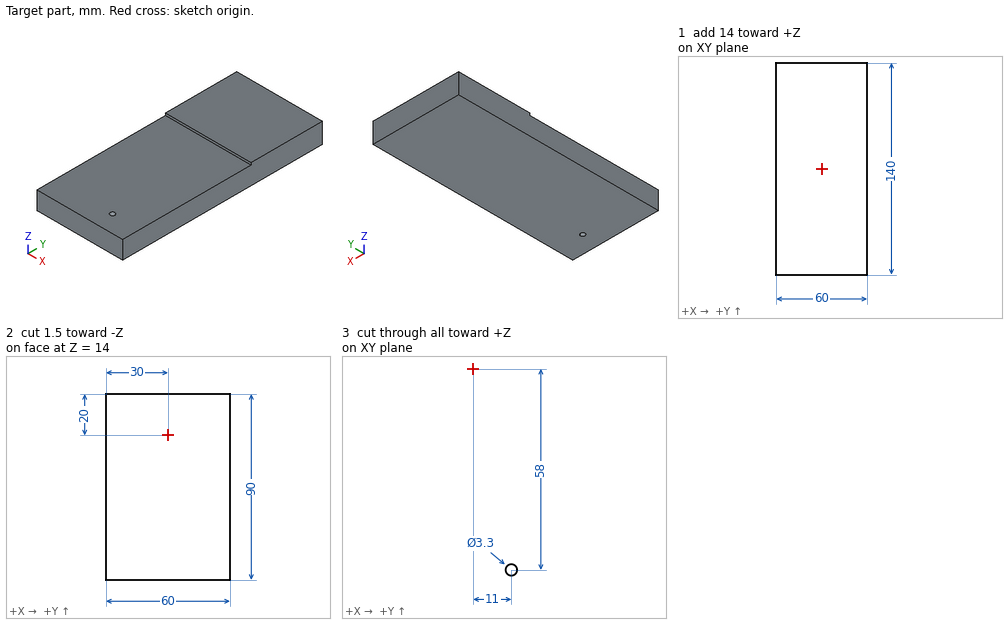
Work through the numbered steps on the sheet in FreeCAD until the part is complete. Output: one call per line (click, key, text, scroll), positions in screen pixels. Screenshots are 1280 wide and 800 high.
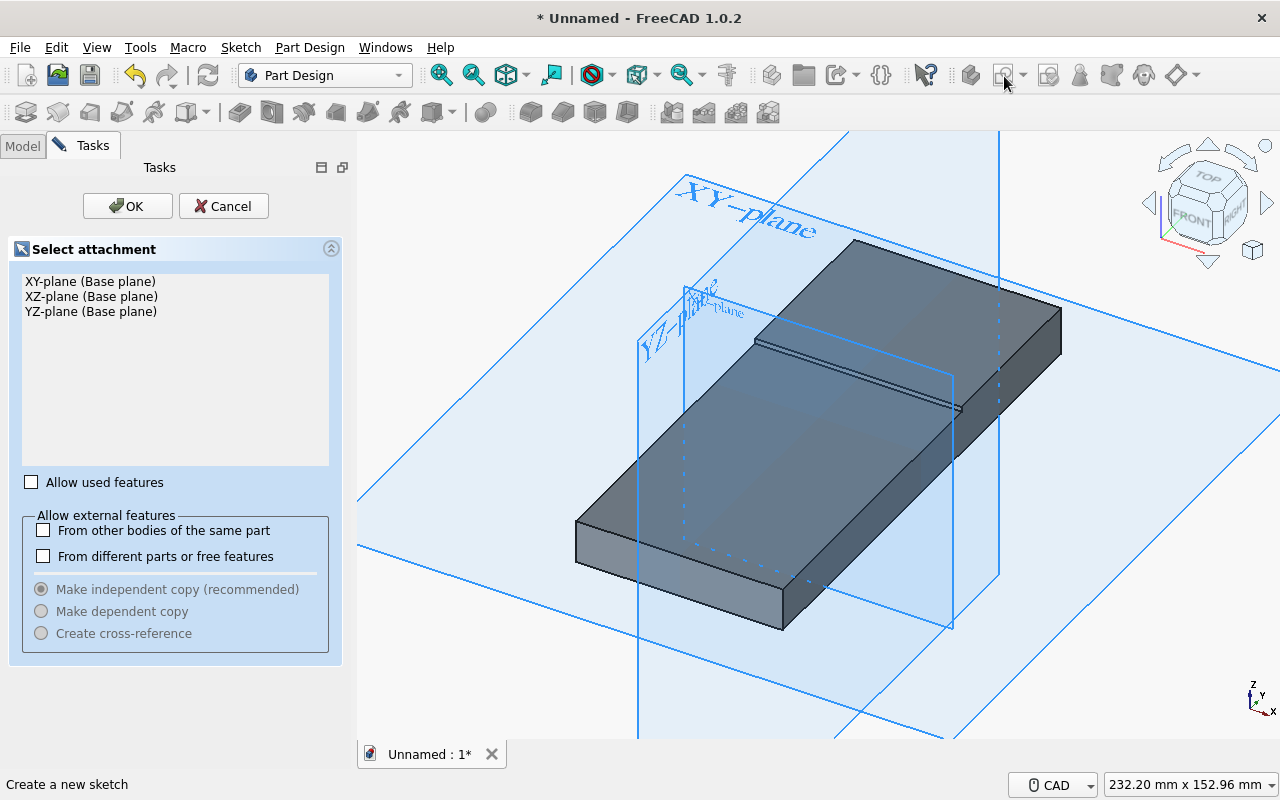
click(82, 282)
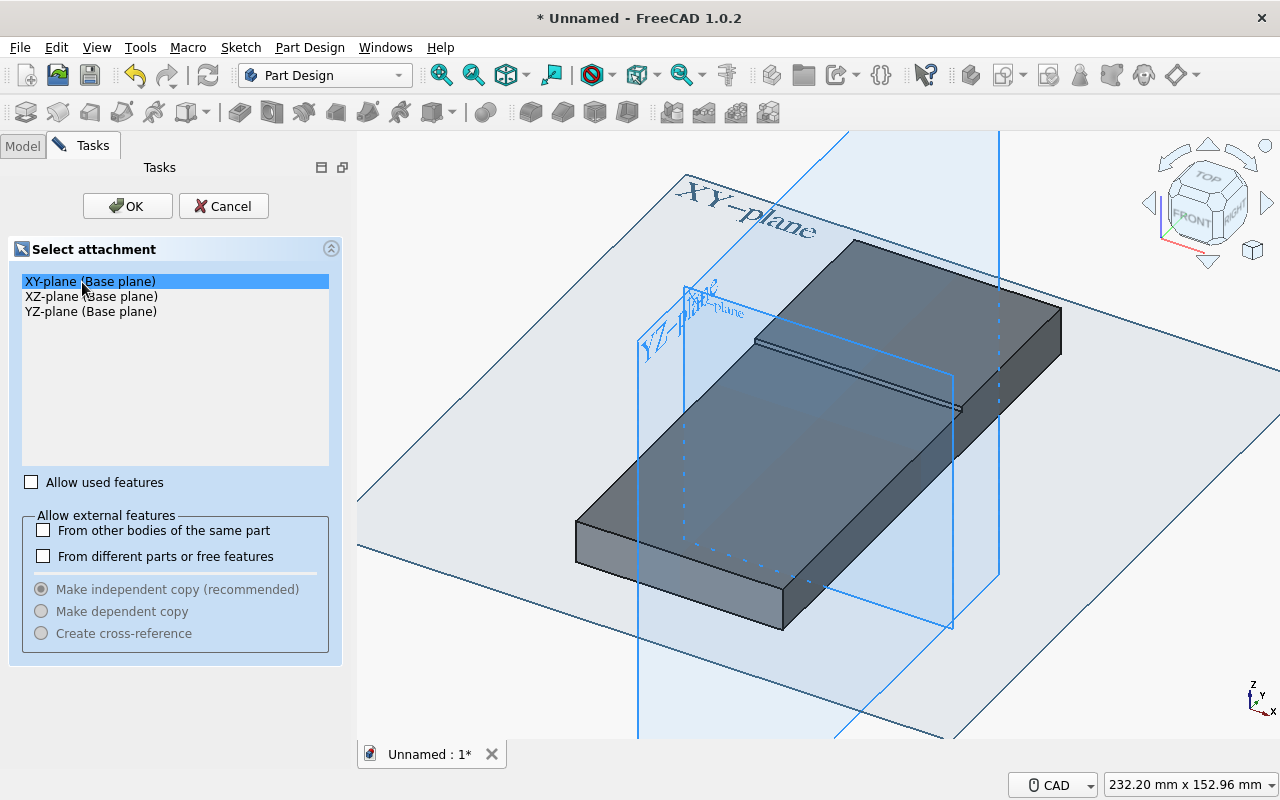
click(128, 206)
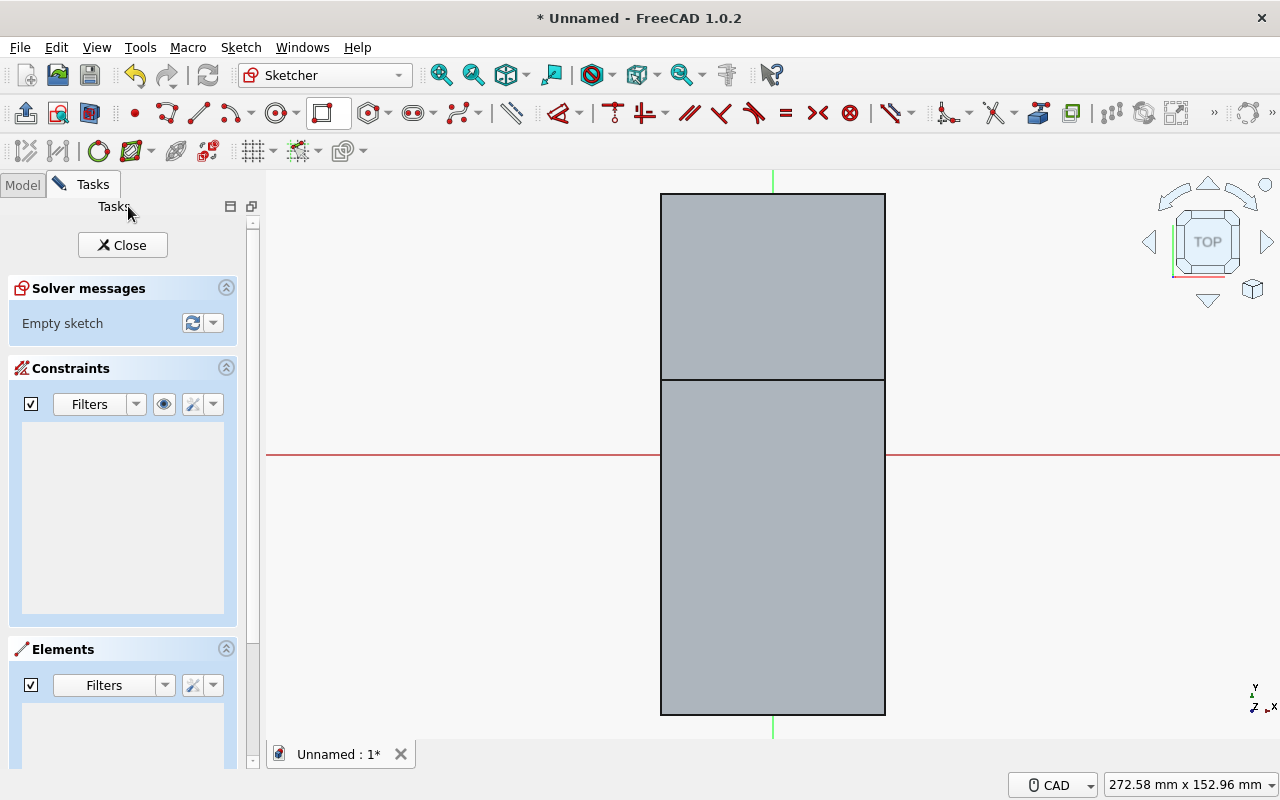
click(90, 114)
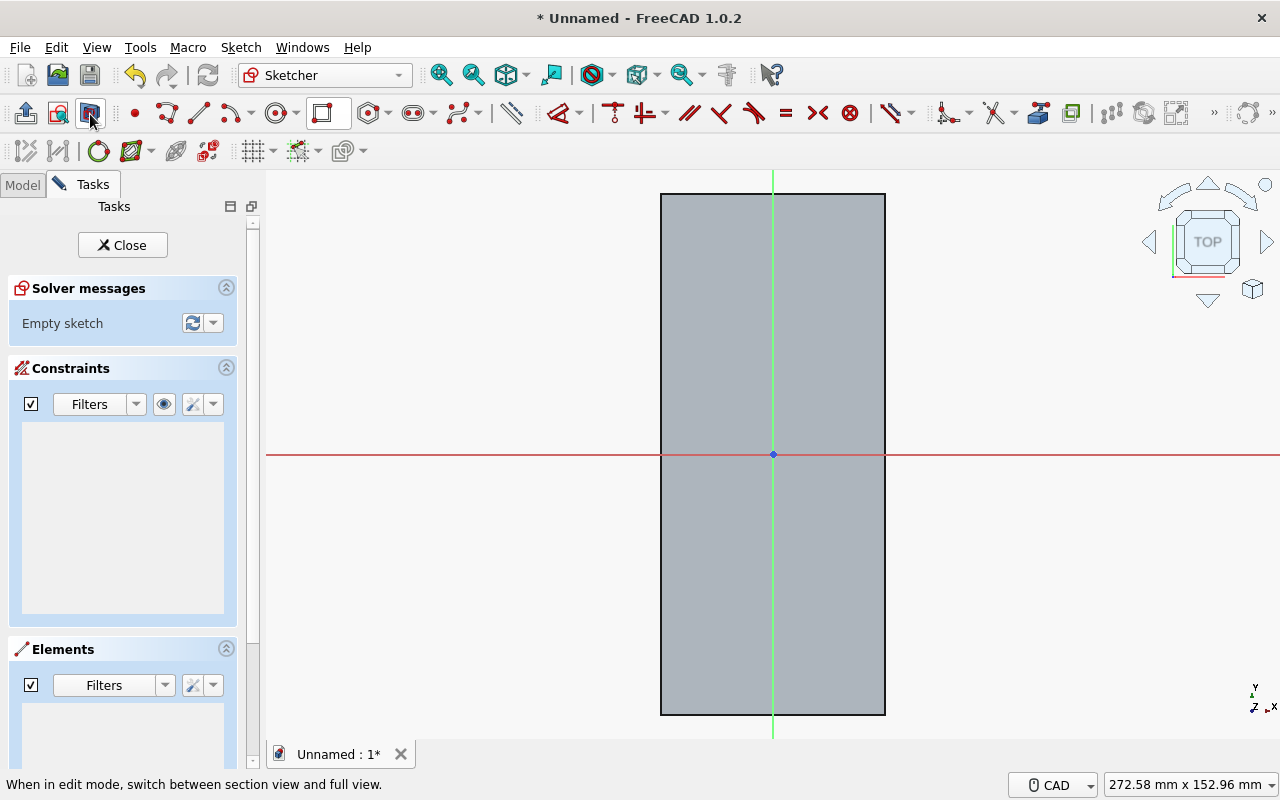
scroll(820, 682, up, 15)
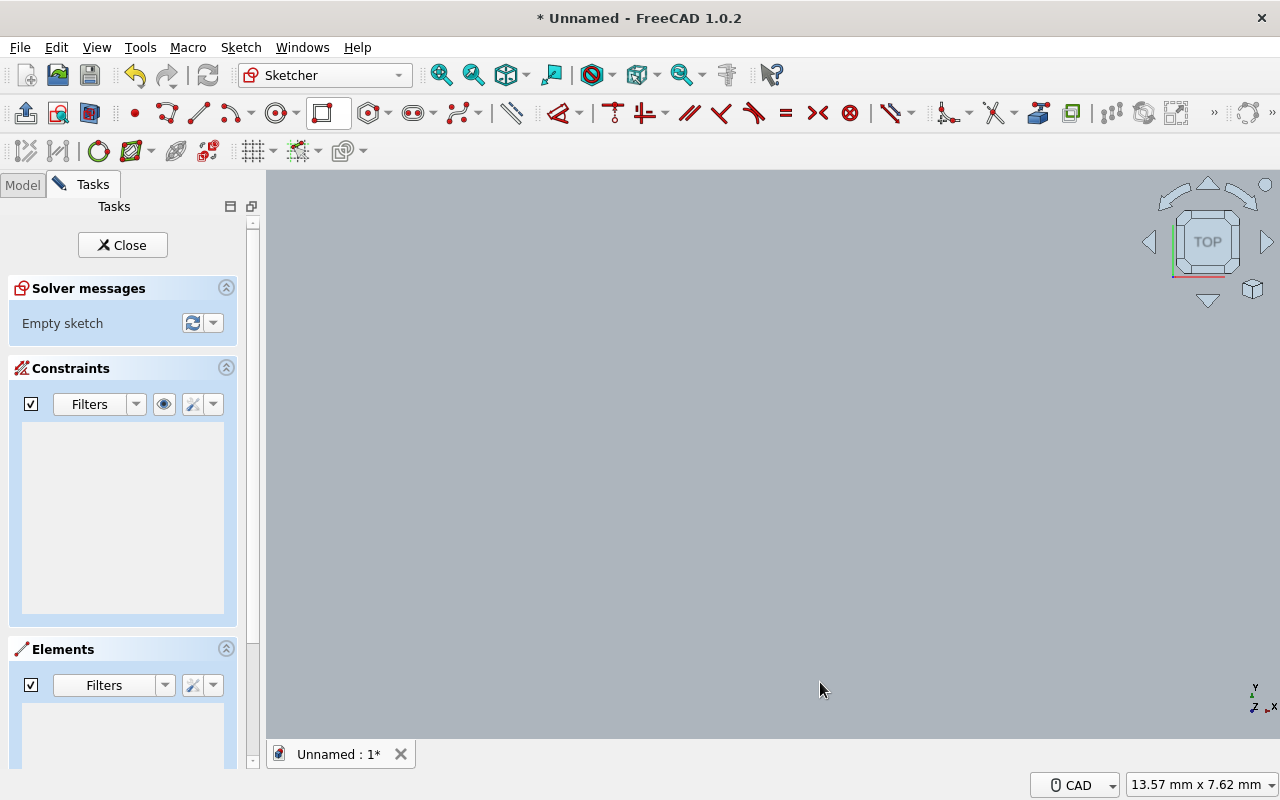
scroll(653, 377, up, 2)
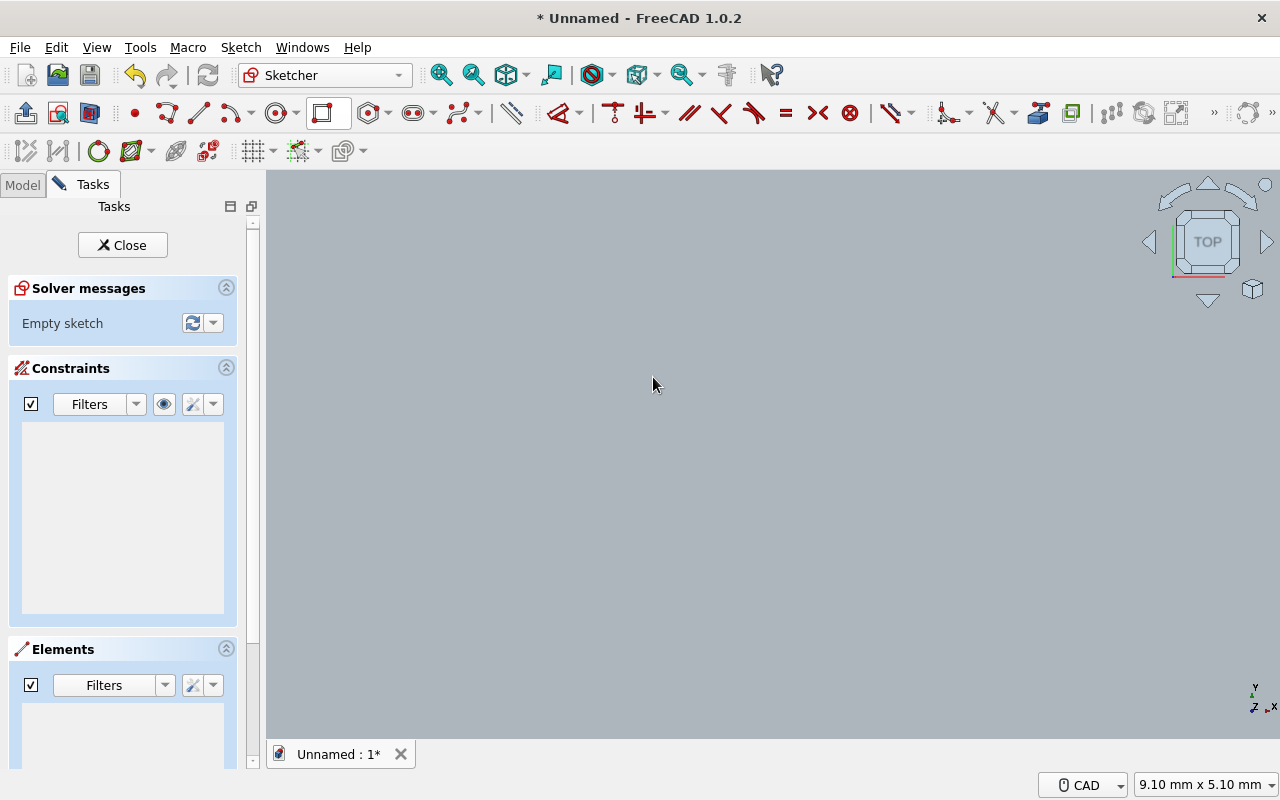
click(276, 114)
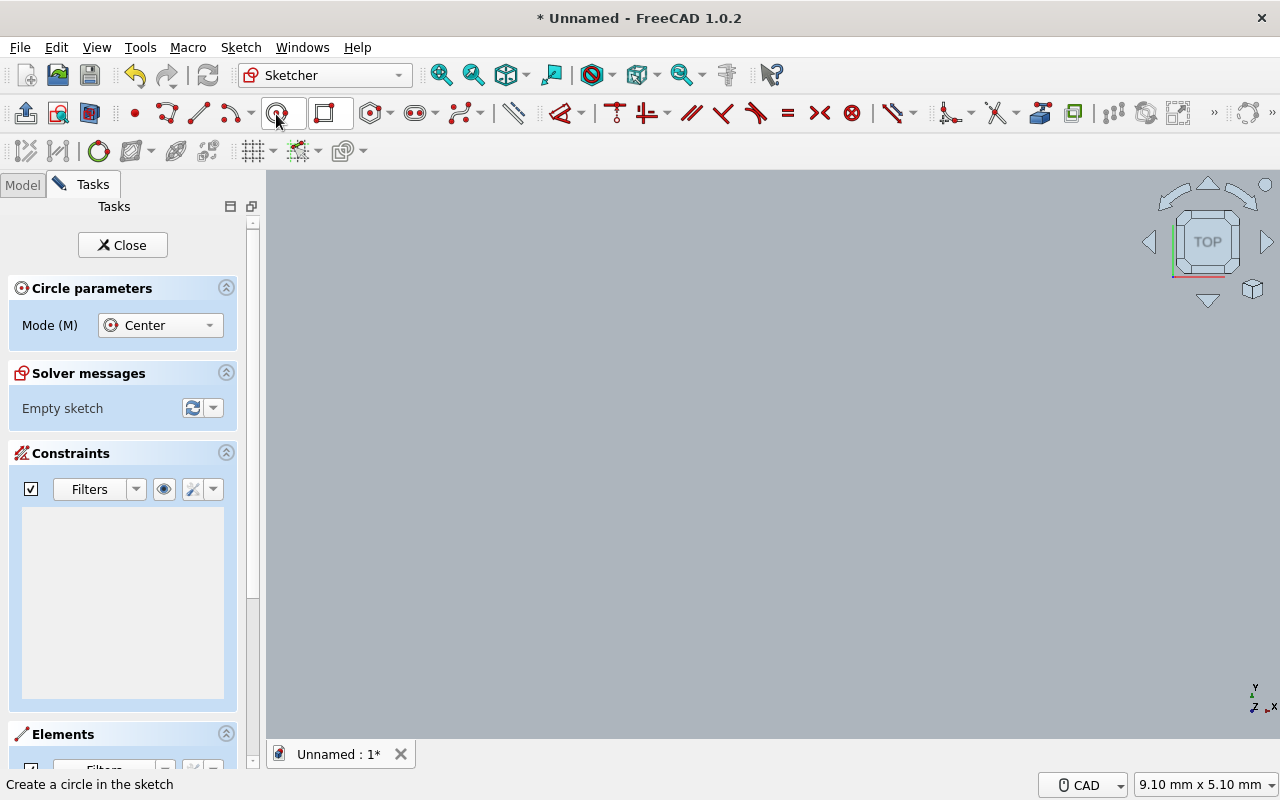
click(704, 454)
move(834, 324)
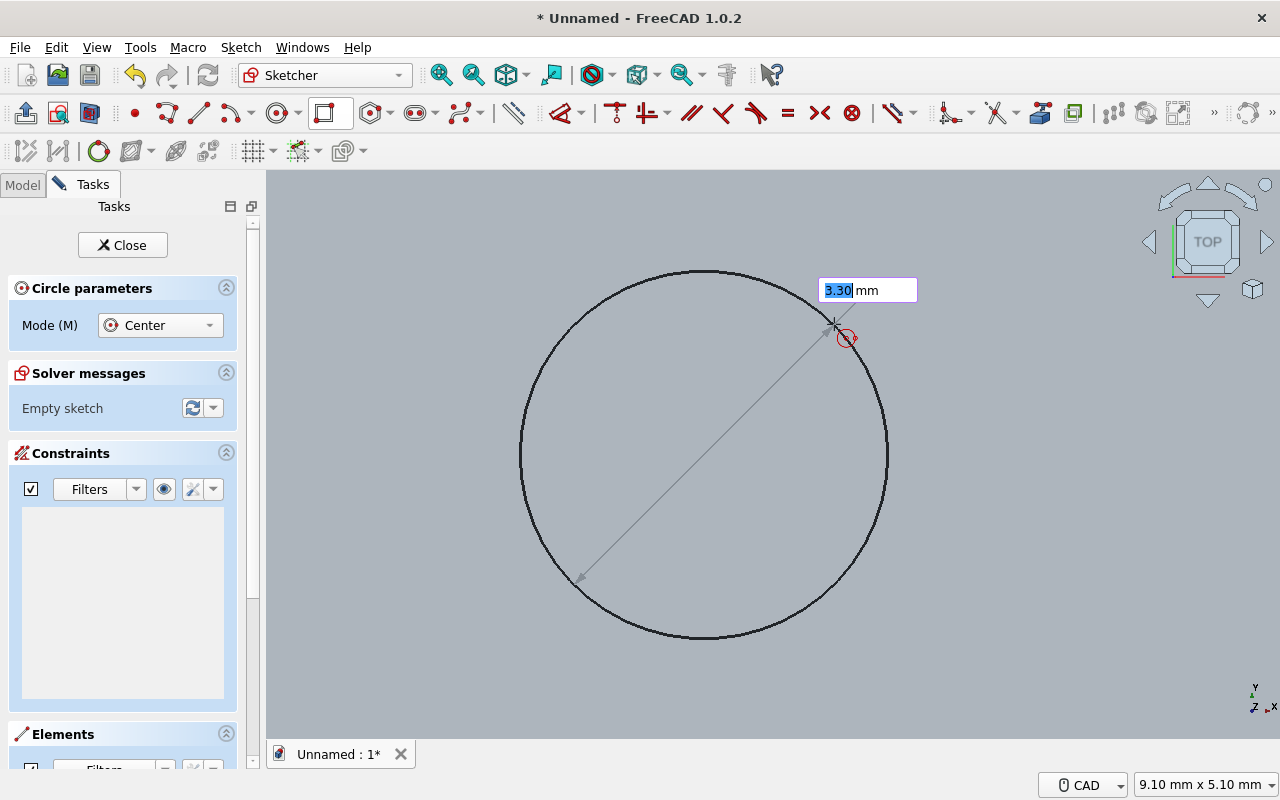
text(3.3)
key(Return)
key(Escape)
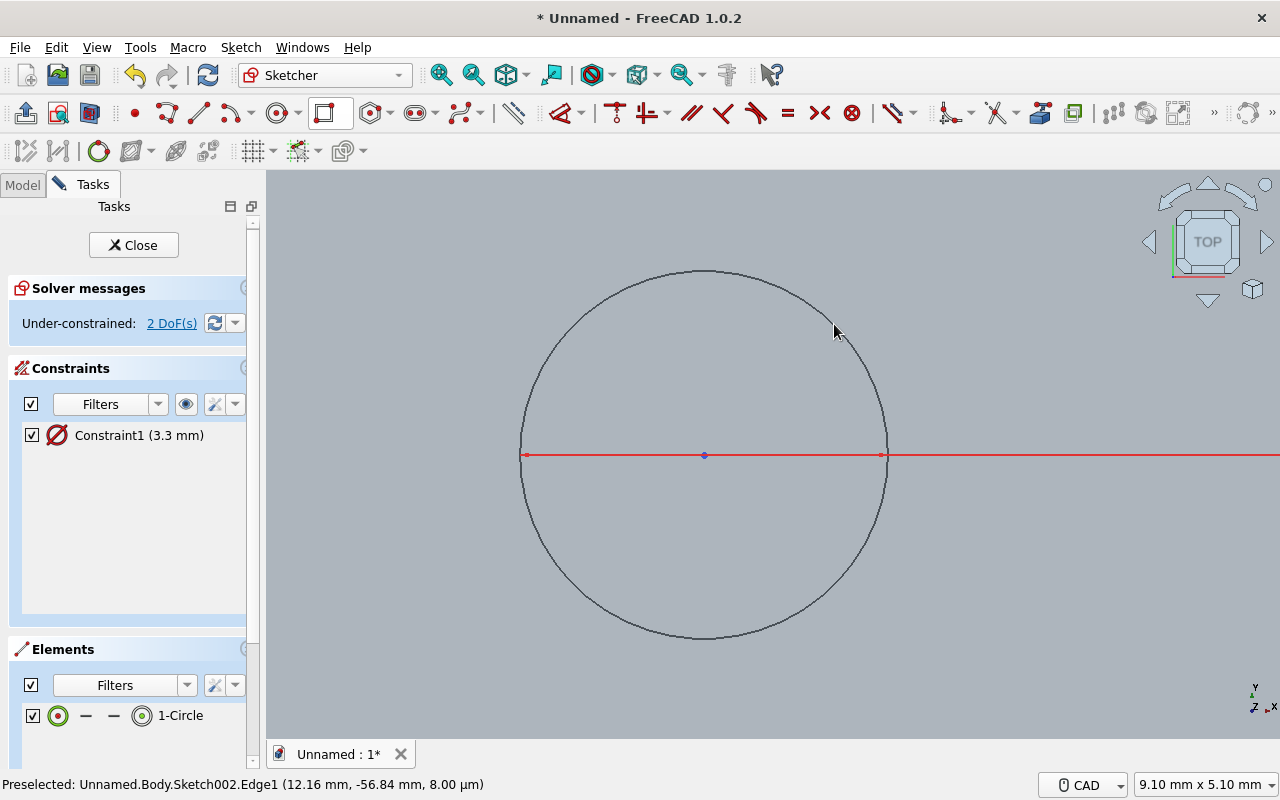
click(560, 114)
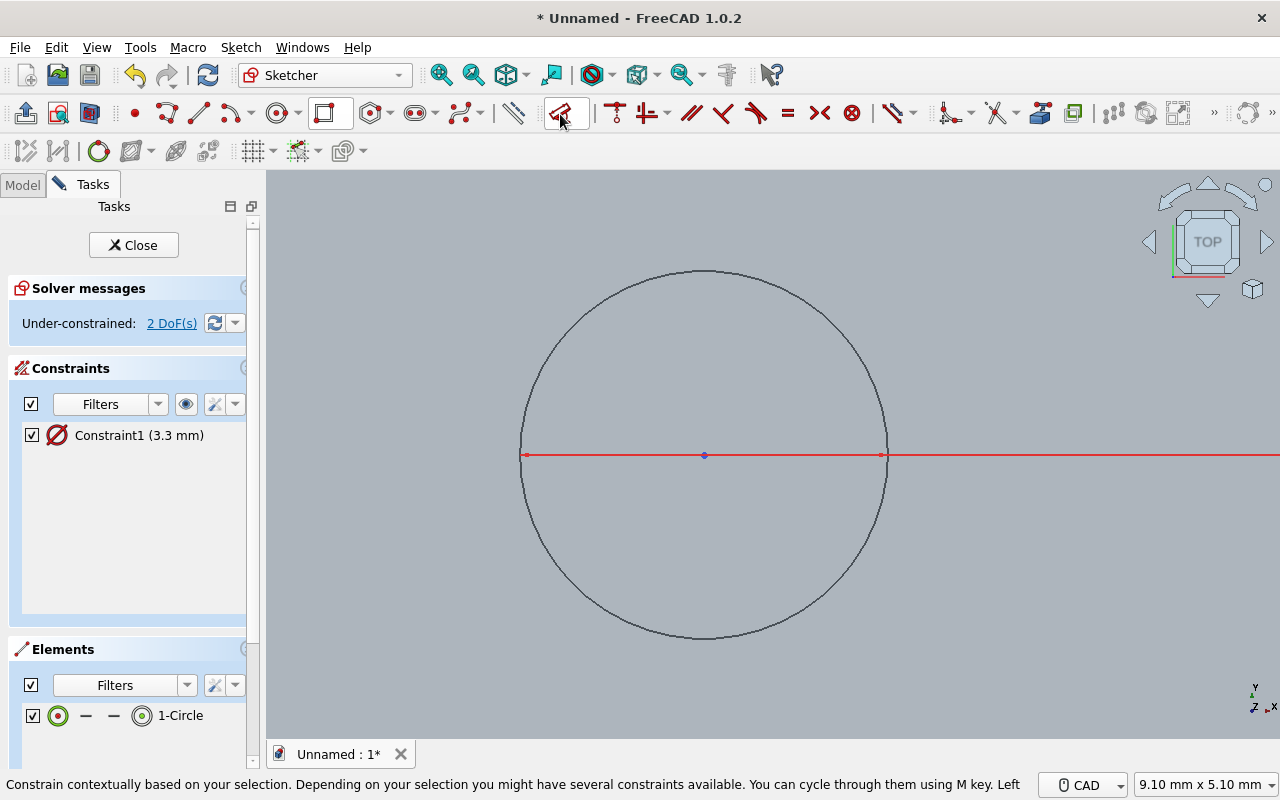
click(704, 455)
click(499, 489)